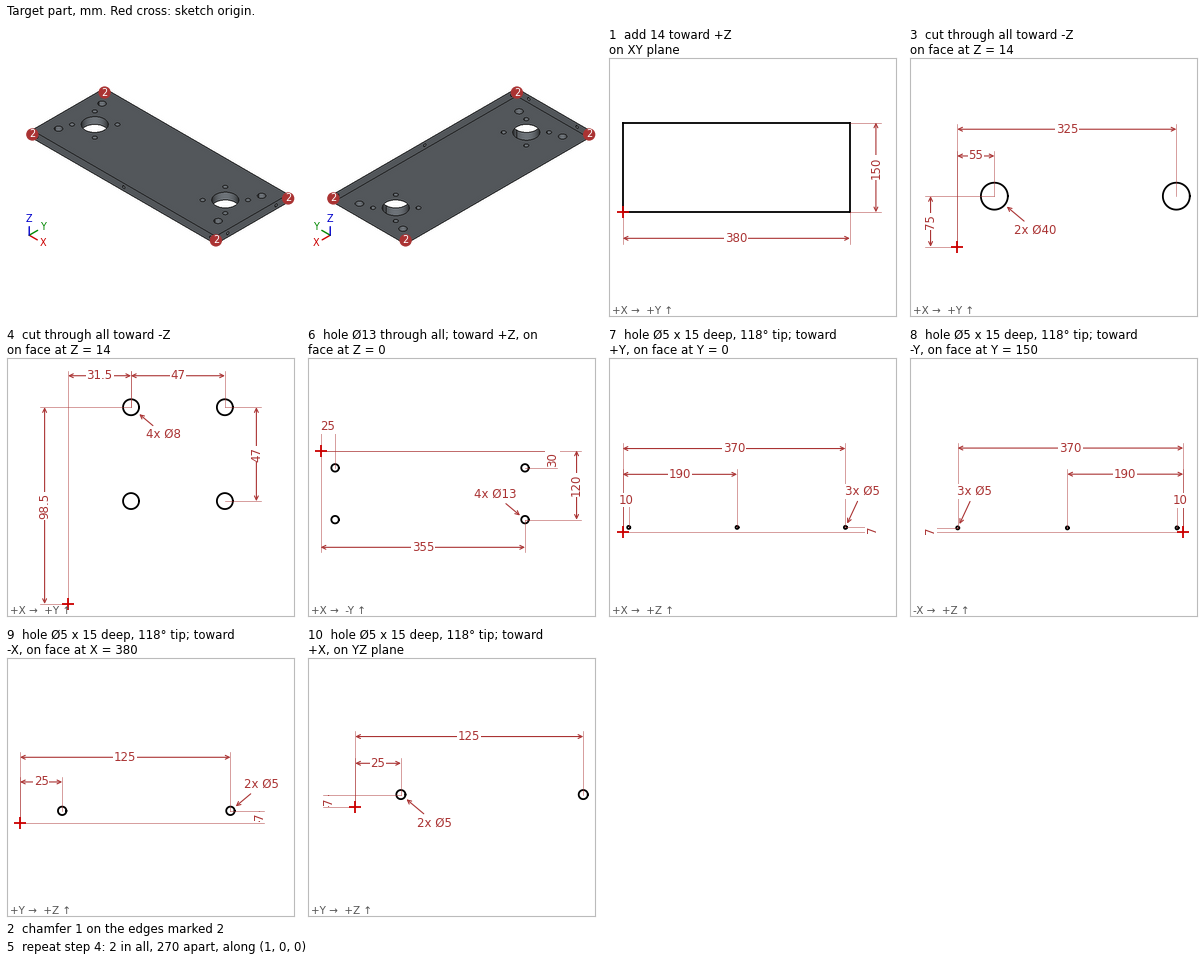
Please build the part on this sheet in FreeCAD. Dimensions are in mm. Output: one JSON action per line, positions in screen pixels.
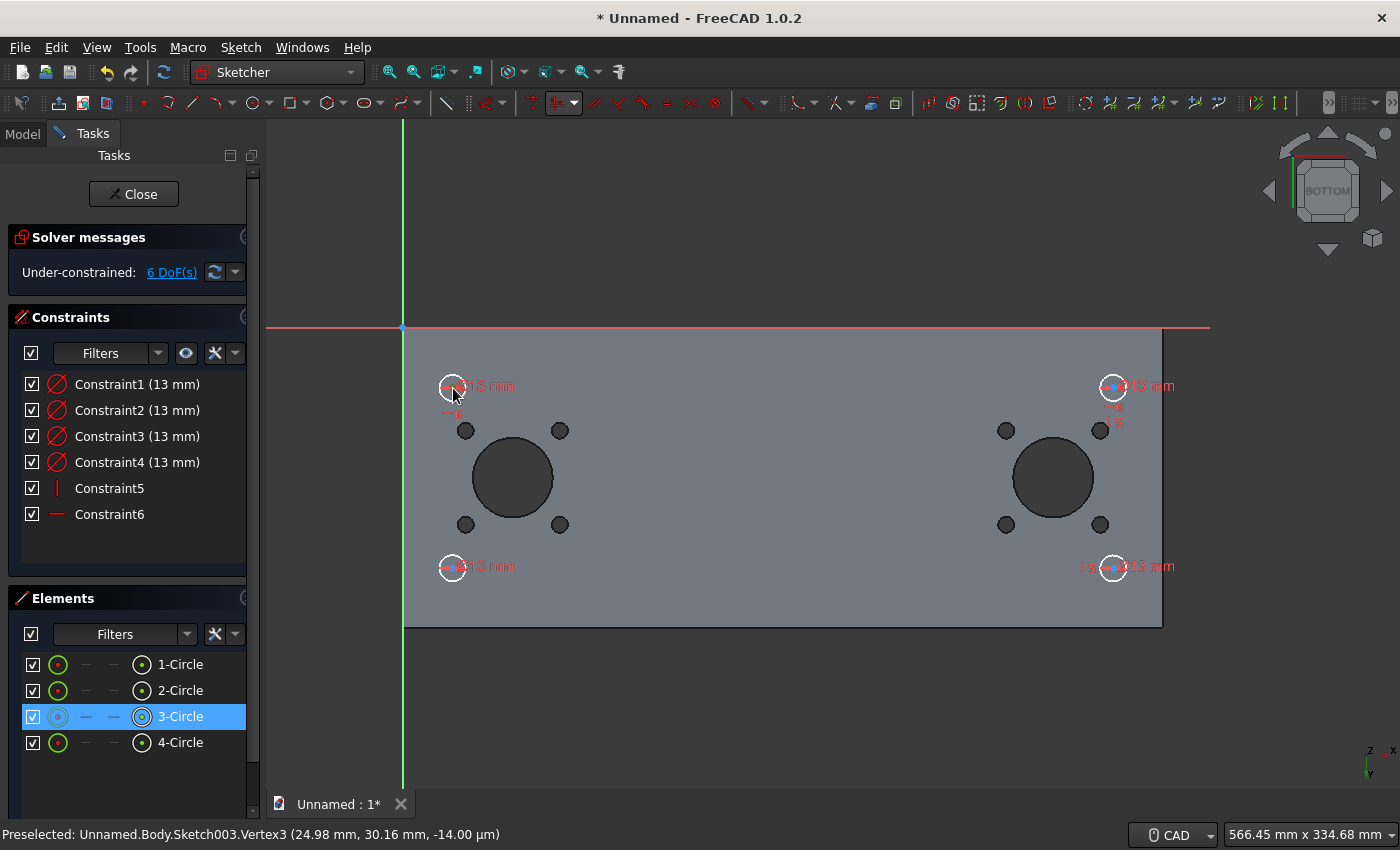
{"action": "left_click", "coordinate": [453, 568]}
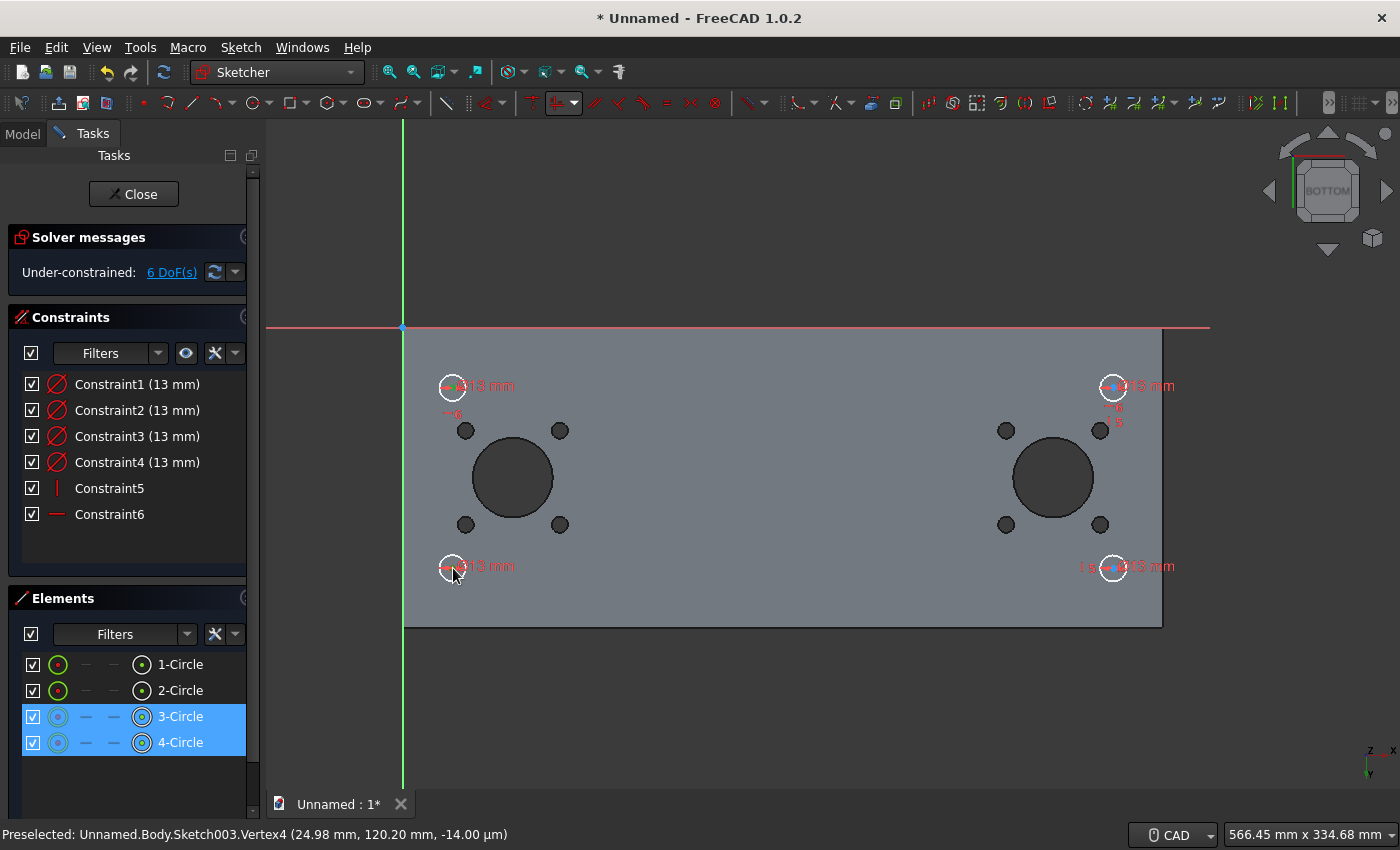
{"action": "key", "text": "v"}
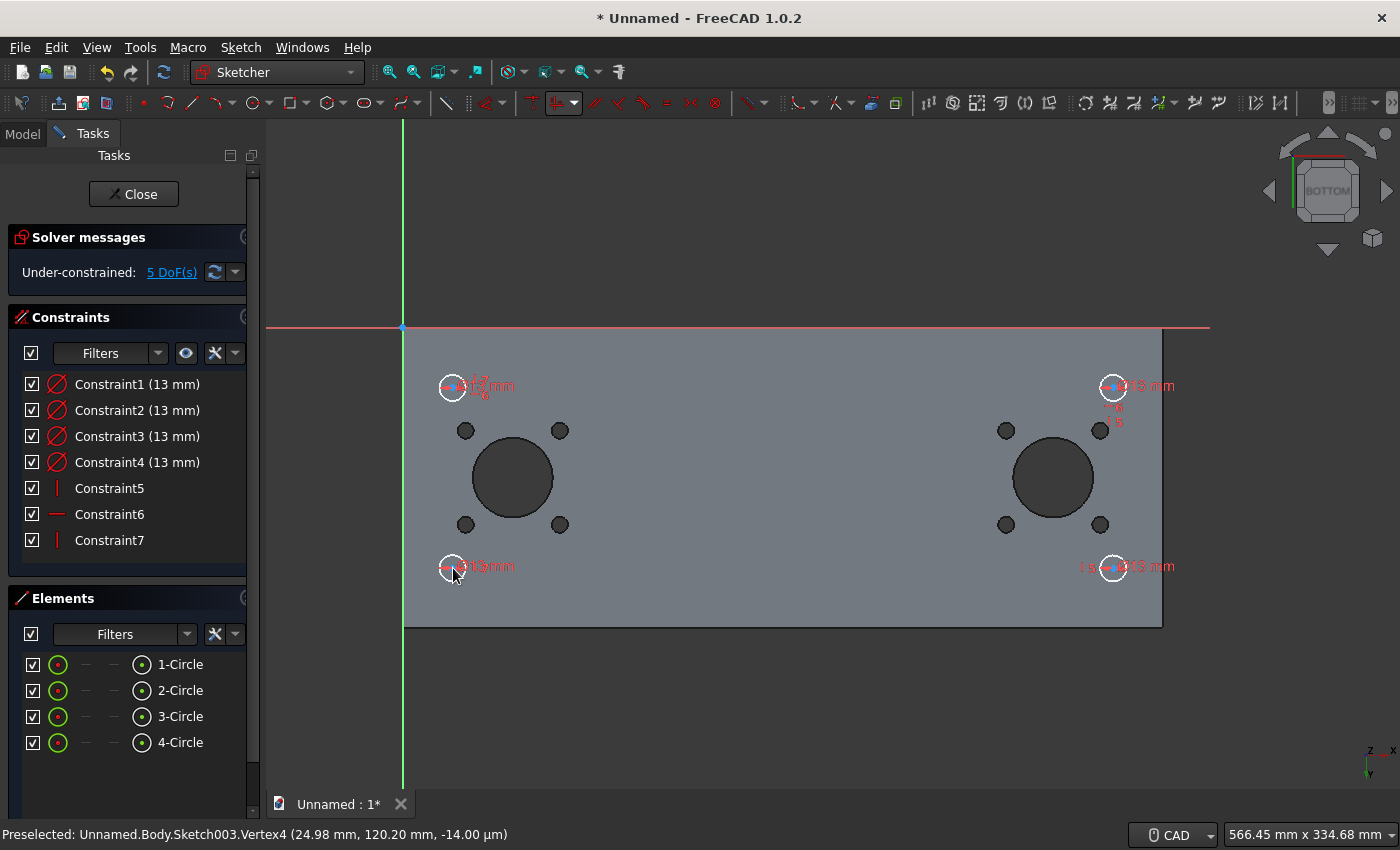
{"action": "left_click", "coordinate": [1113, 568]}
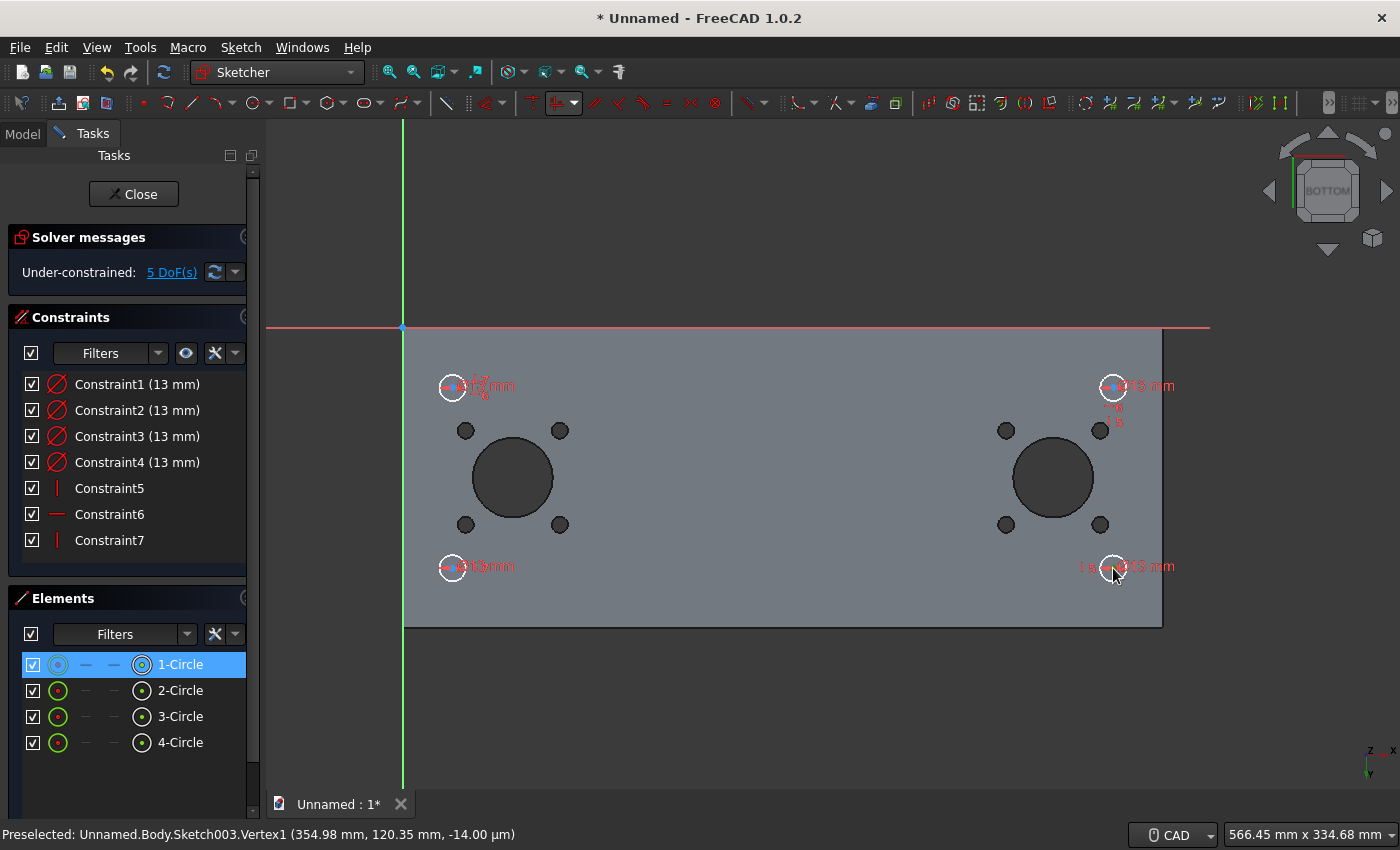
{"action": "left_click", "coordinate": [453, 568]}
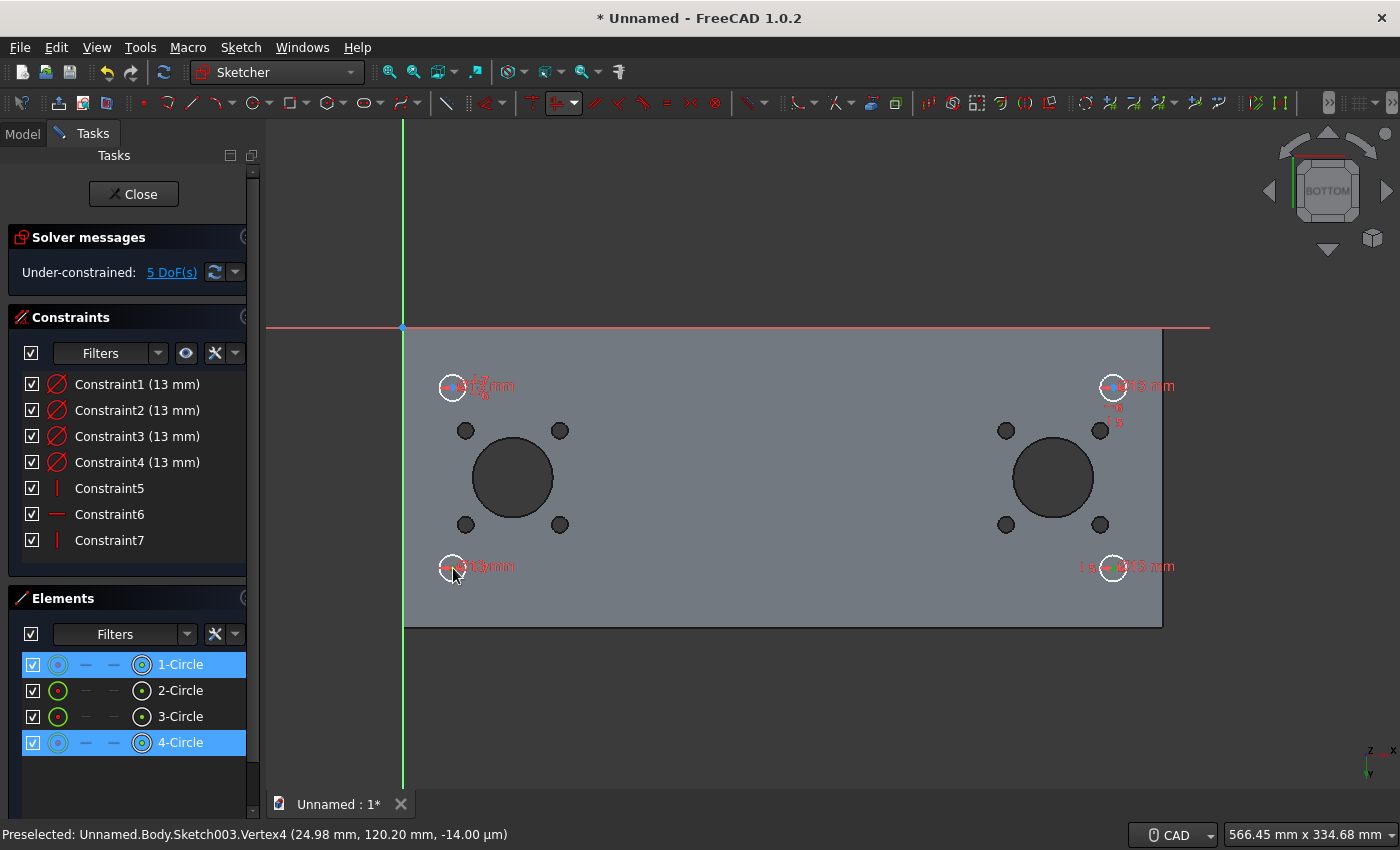
{"action": "key", "text": "h"}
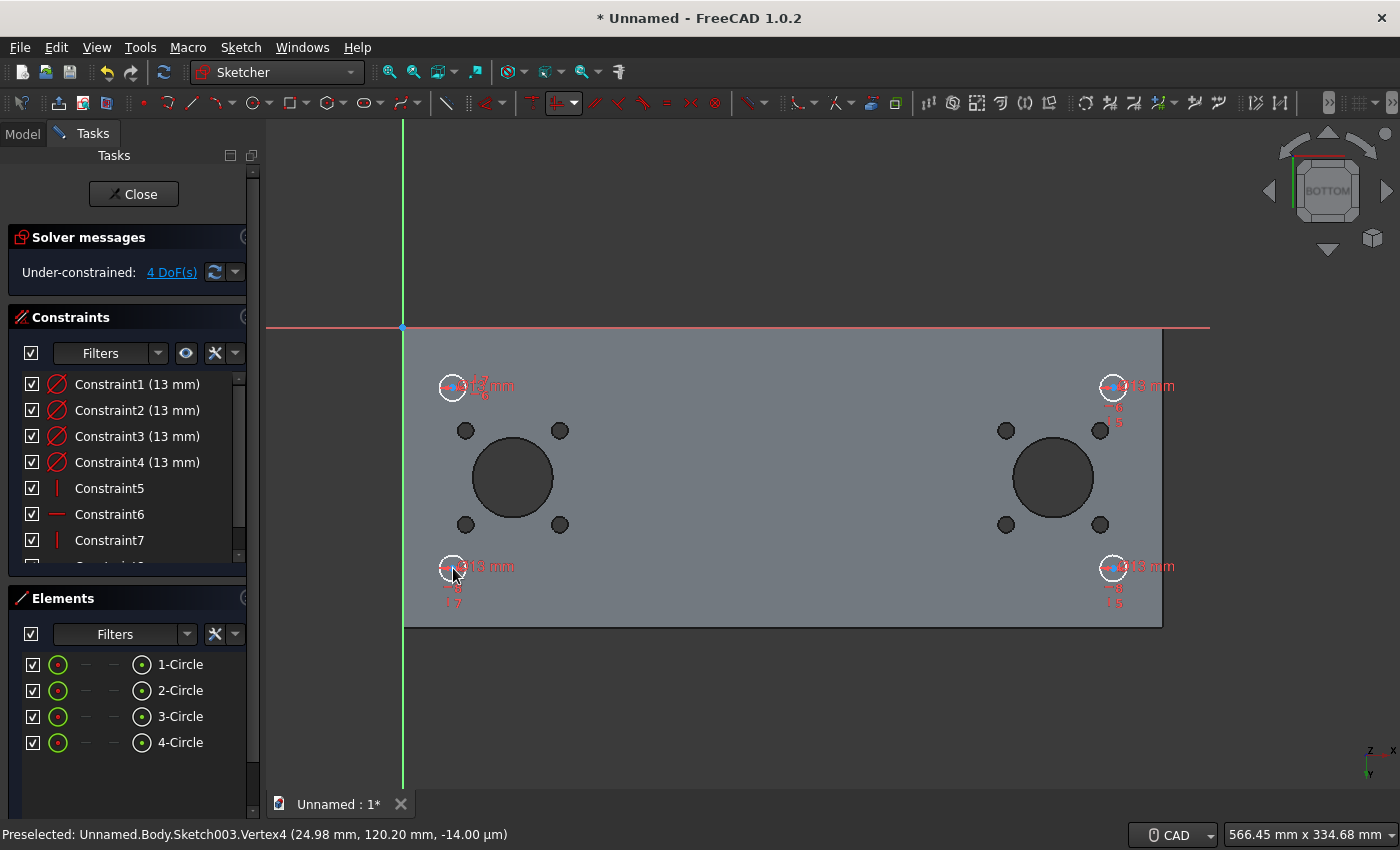
{"action": "left_click", "coordinate": [486, 104]}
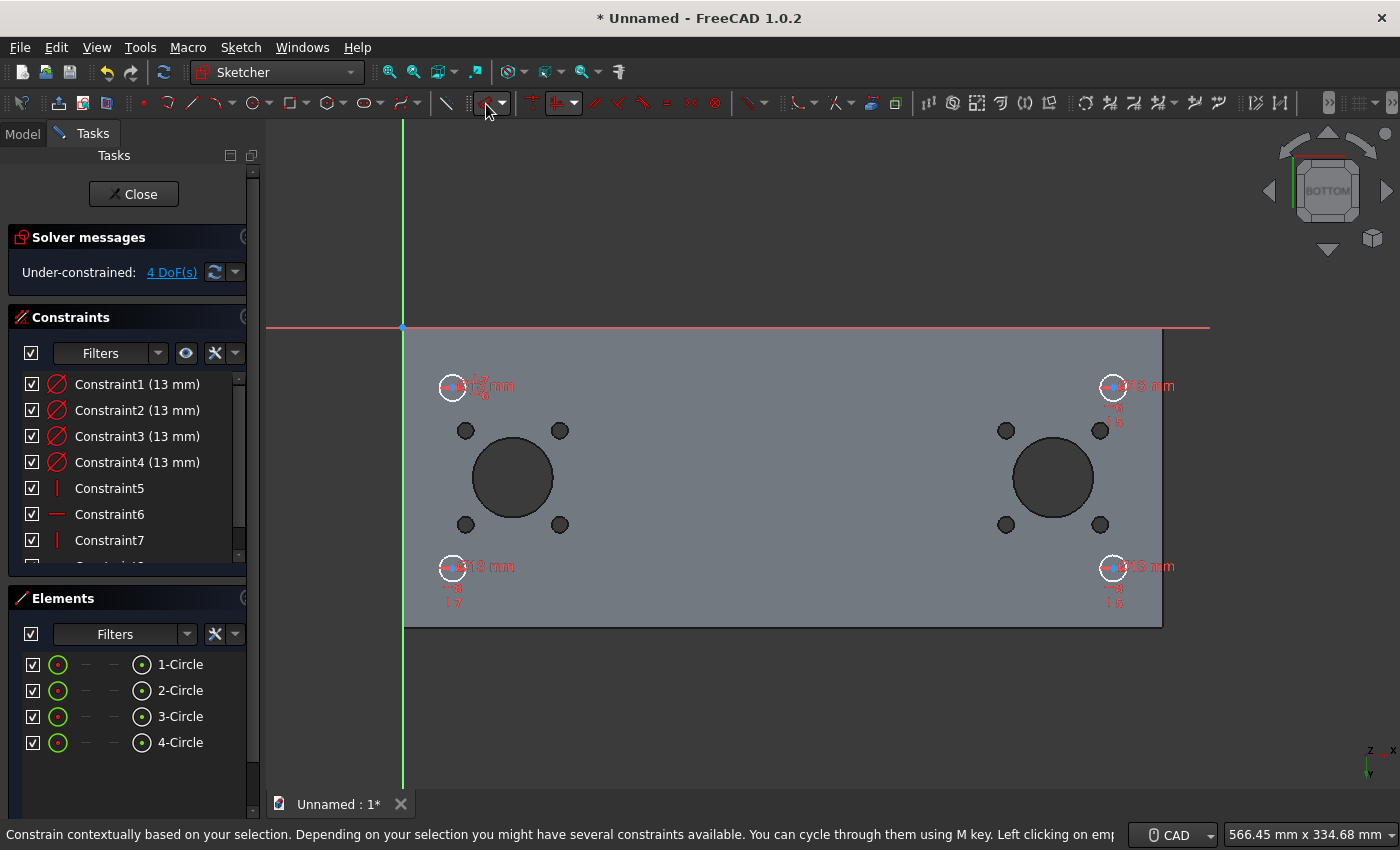
{"action": "left_click", "coordinate": [1113, 388]}
{"action": "left_click", "coordinate": [369, 358]}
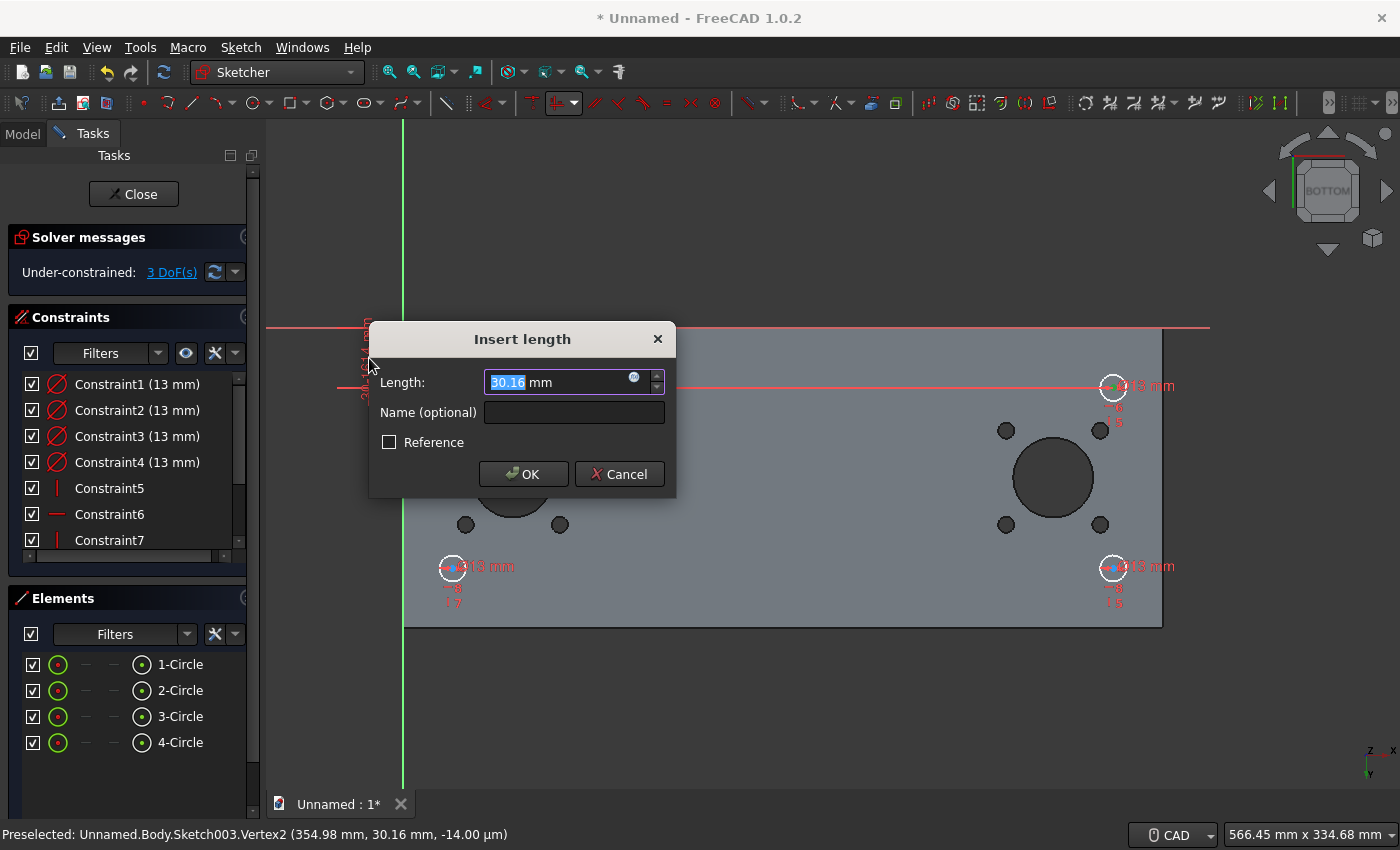
{"action": "type", "text": "30"}
{"action": "key", "text": "Return"}